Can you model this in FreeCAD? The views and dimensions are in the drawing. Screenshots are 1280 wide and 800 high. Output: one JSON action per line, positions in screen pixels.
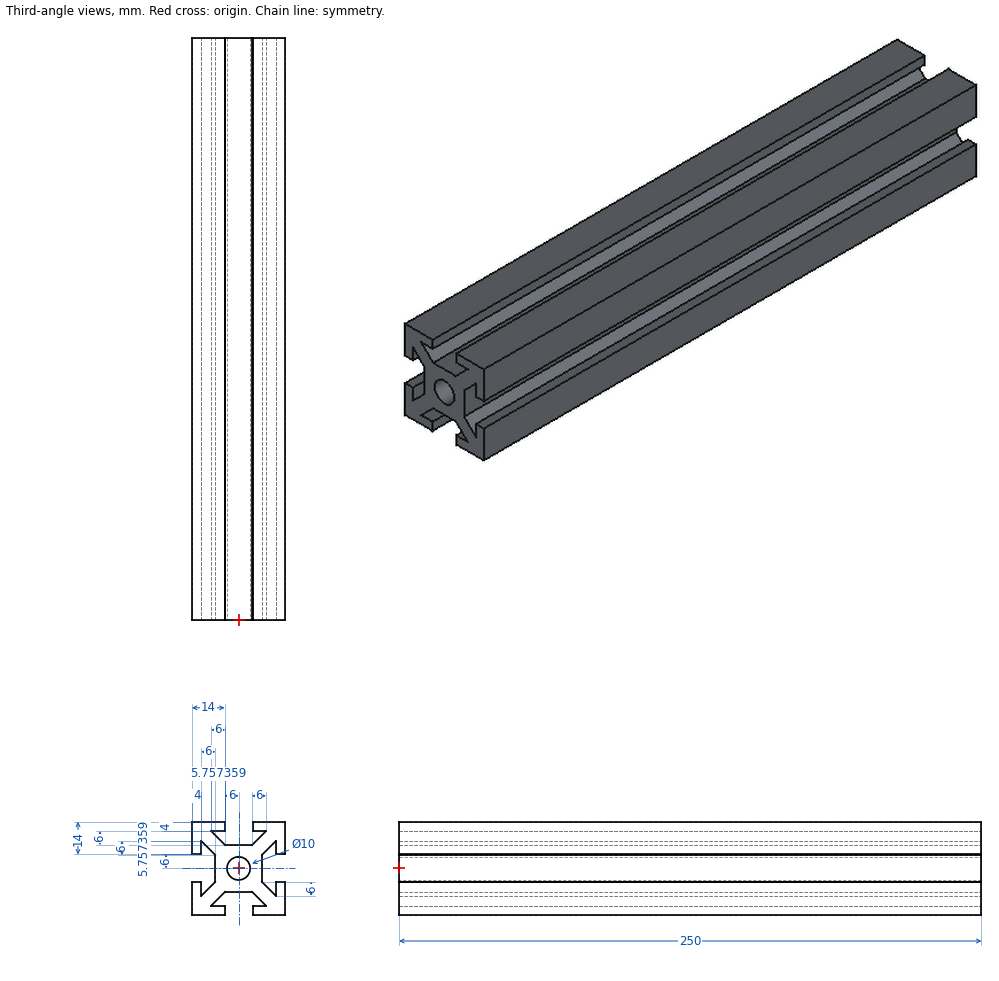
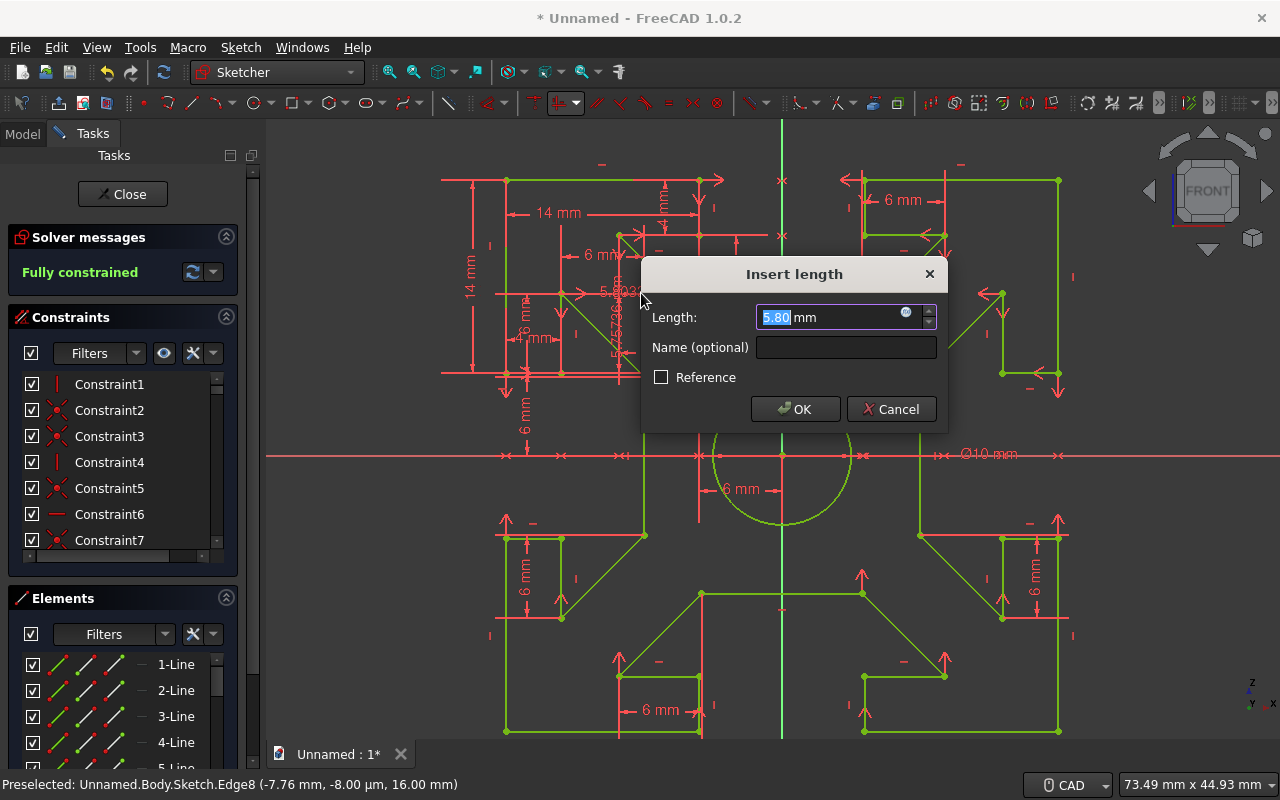
{"action": "type", "text": "5.757359"}
{"action": "key", "text": "Return"}
{"action": "key", "text": "Escape"}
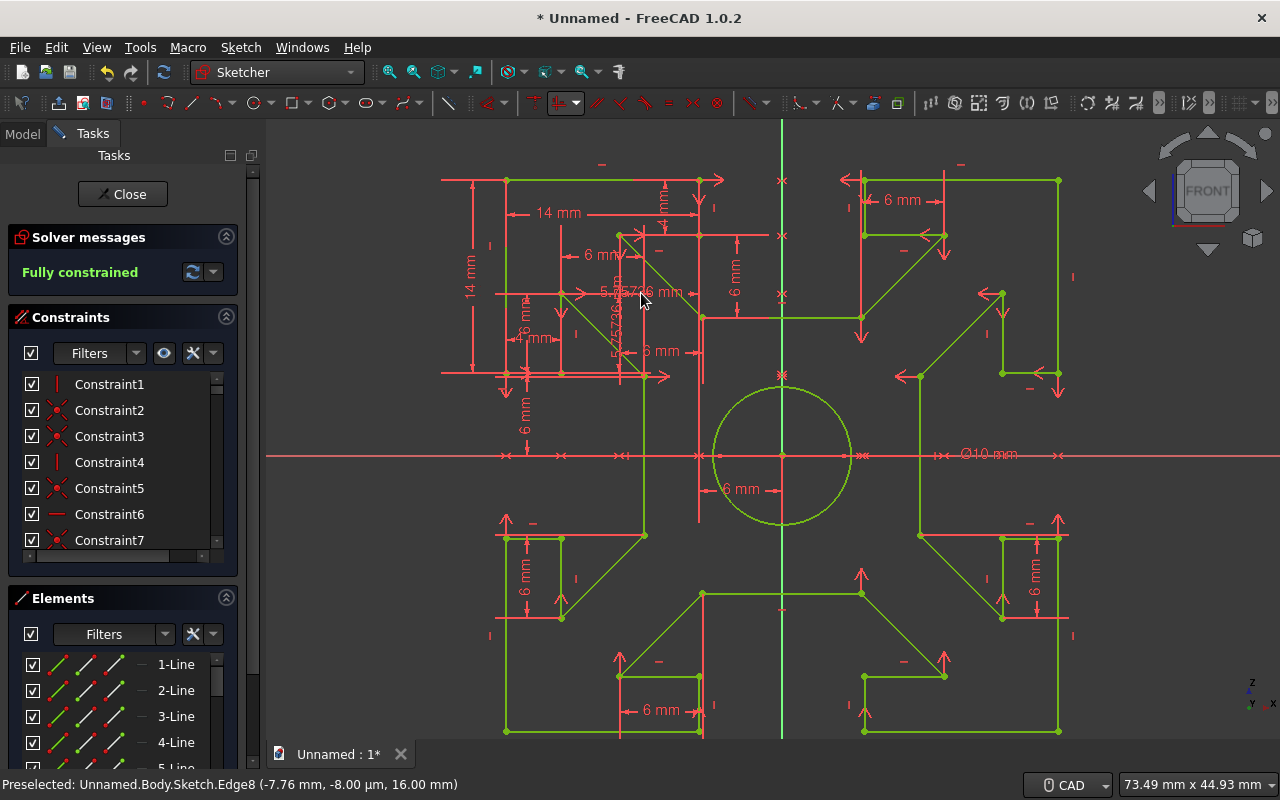
{"action": "left_click", "coordinate": [123, 194]}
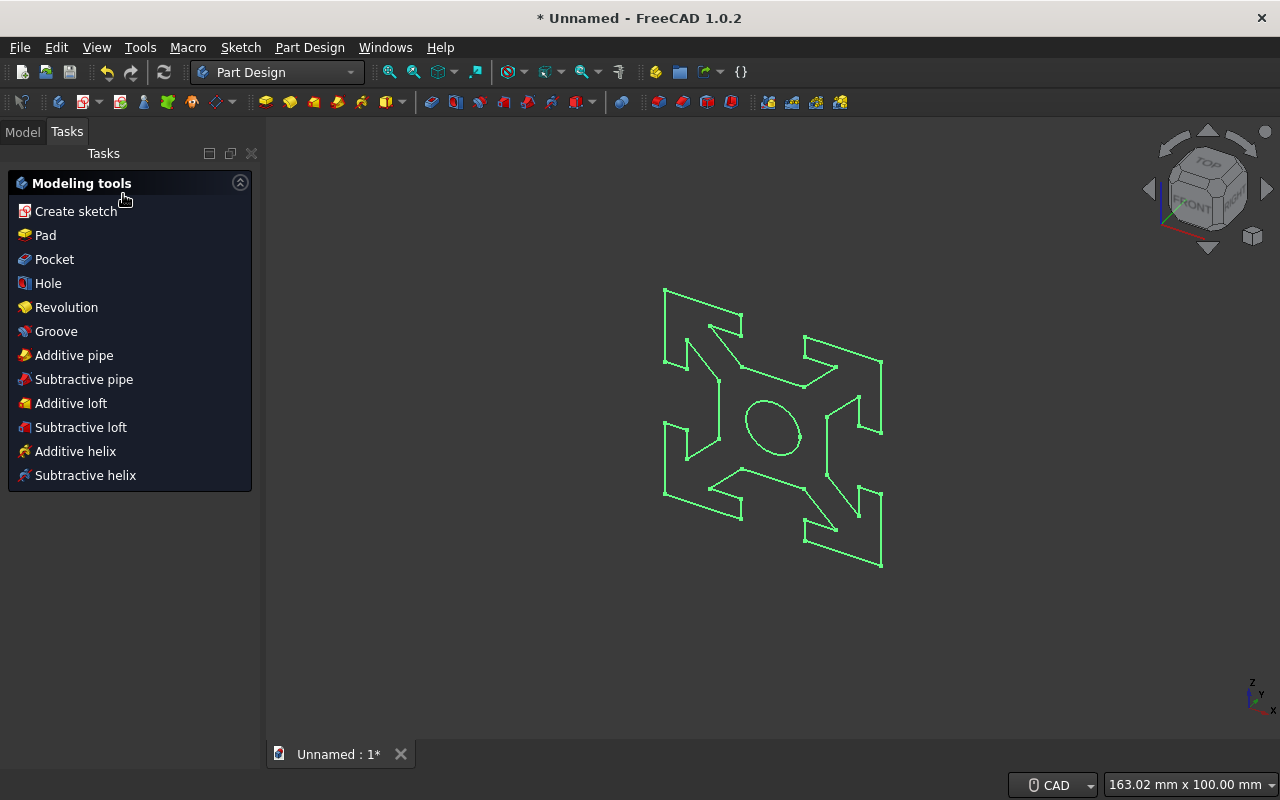
{"action": "left_click", "coordinate": [266, 102]}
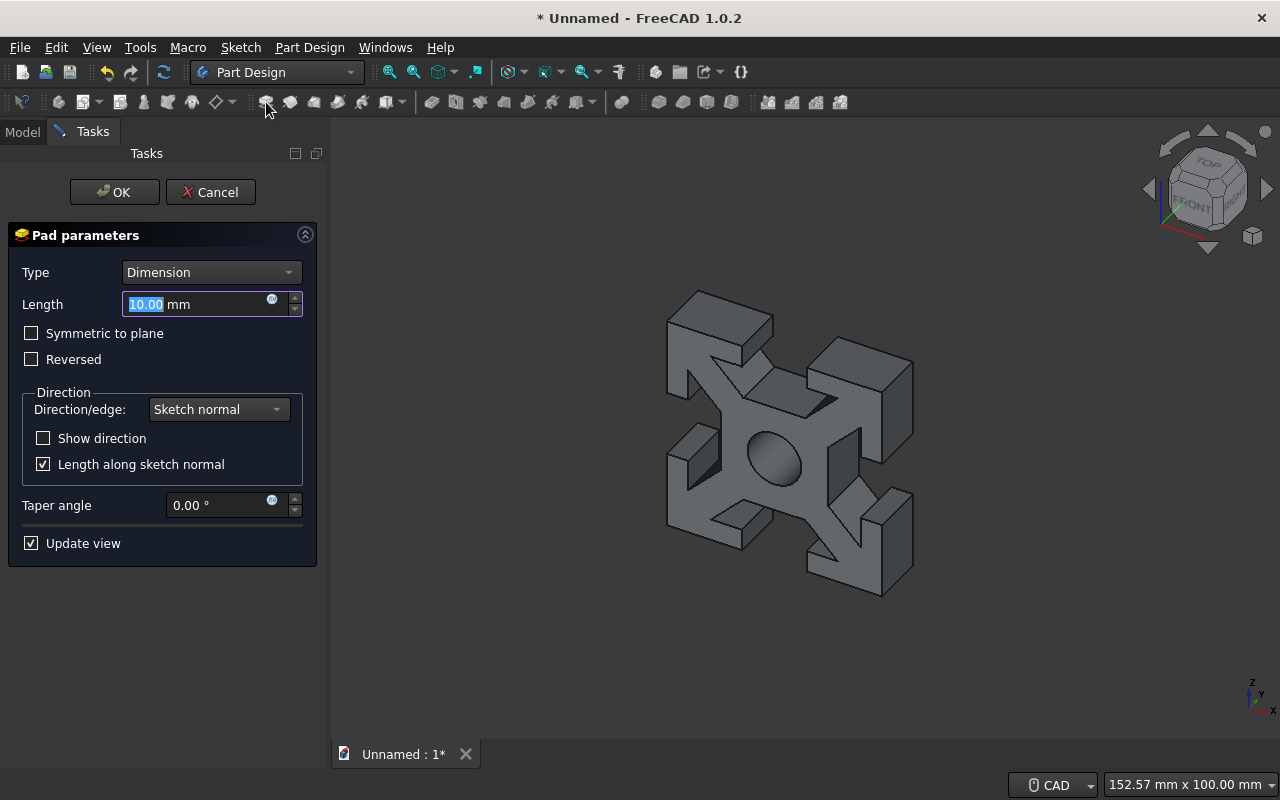
{"action": "type", "text": "250"}
{"action": "key", "text": "Tab"}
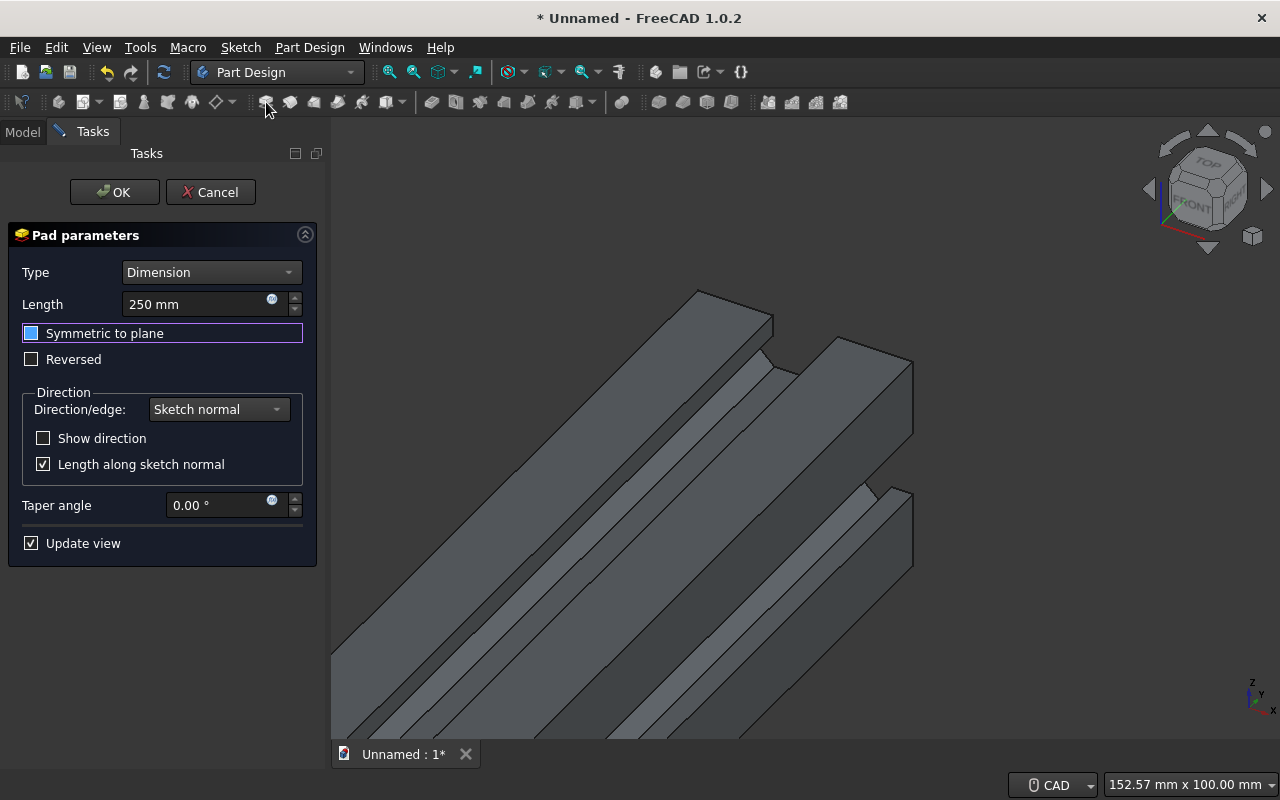
{"action": "left_click", "coordinate": [30, 359]}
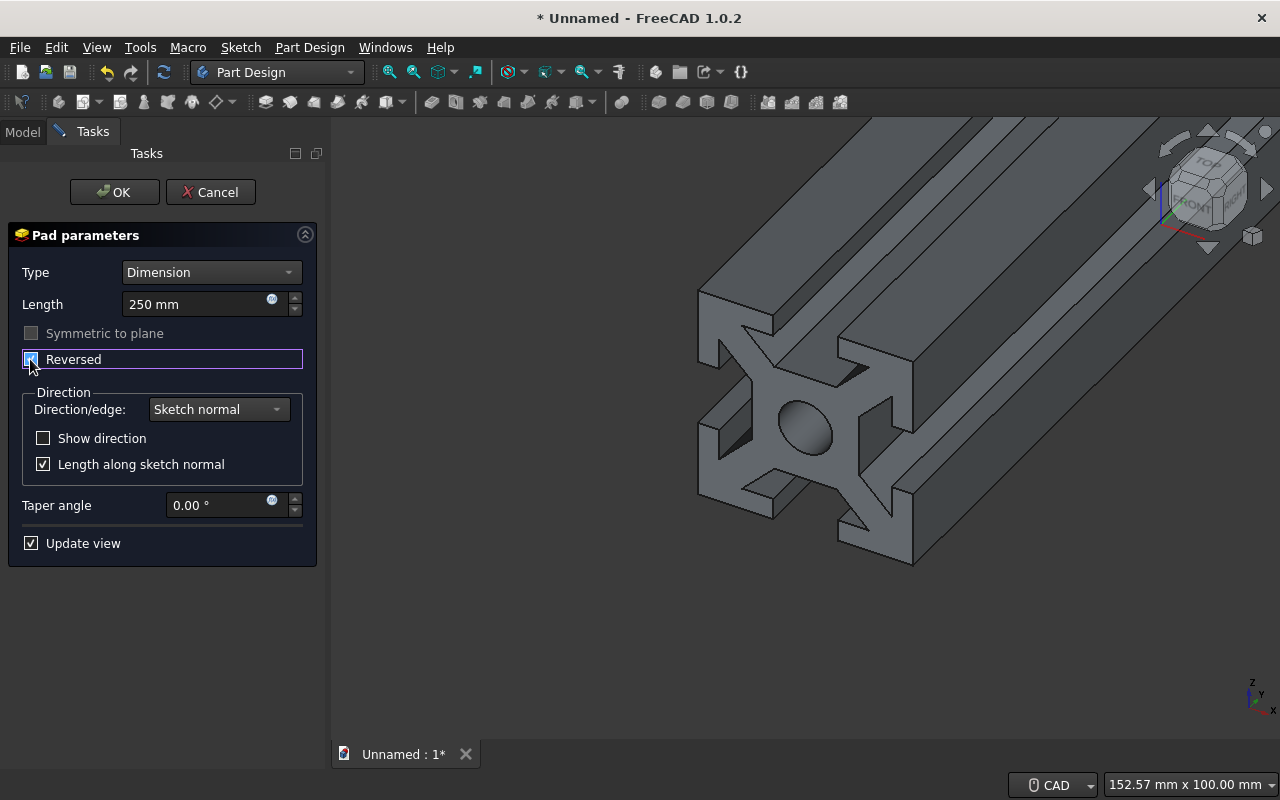
{"action": "left_click", "coordinate": [115, 192]}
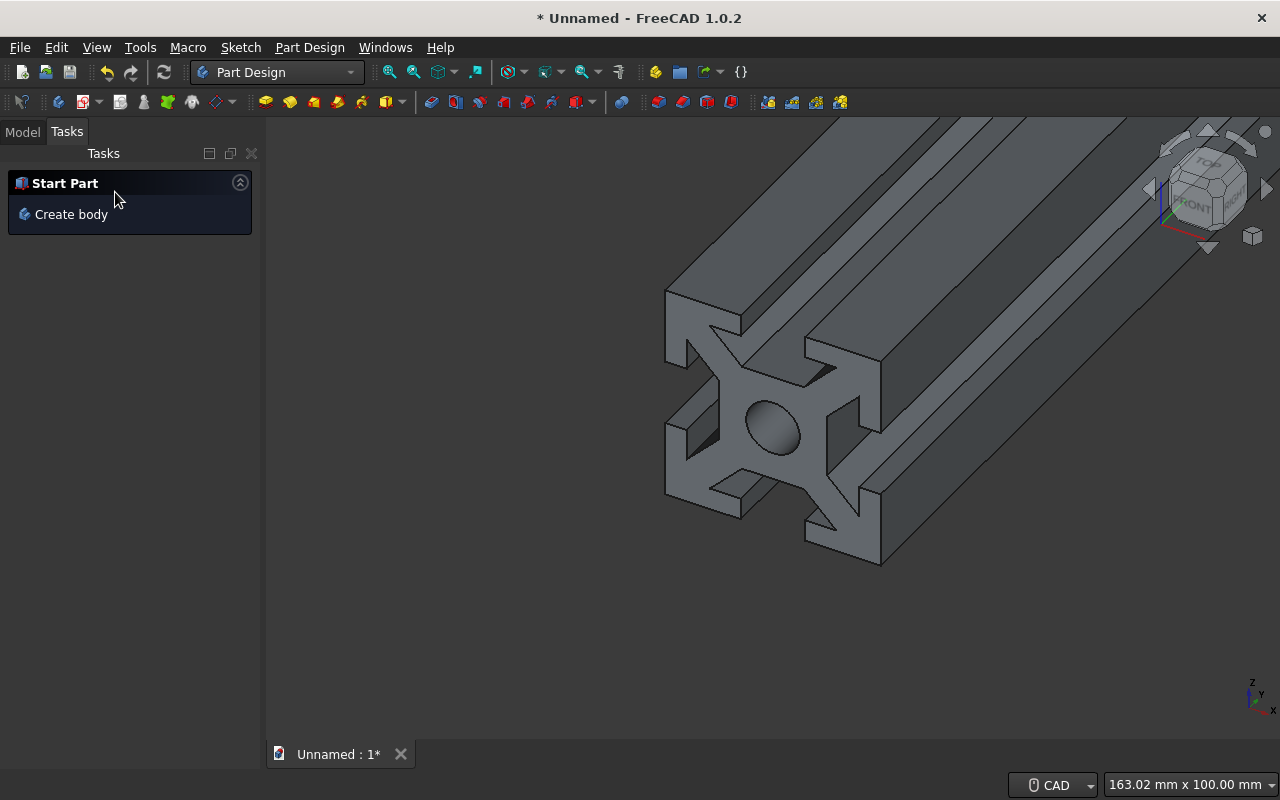
{"action": "key", "text": "0"}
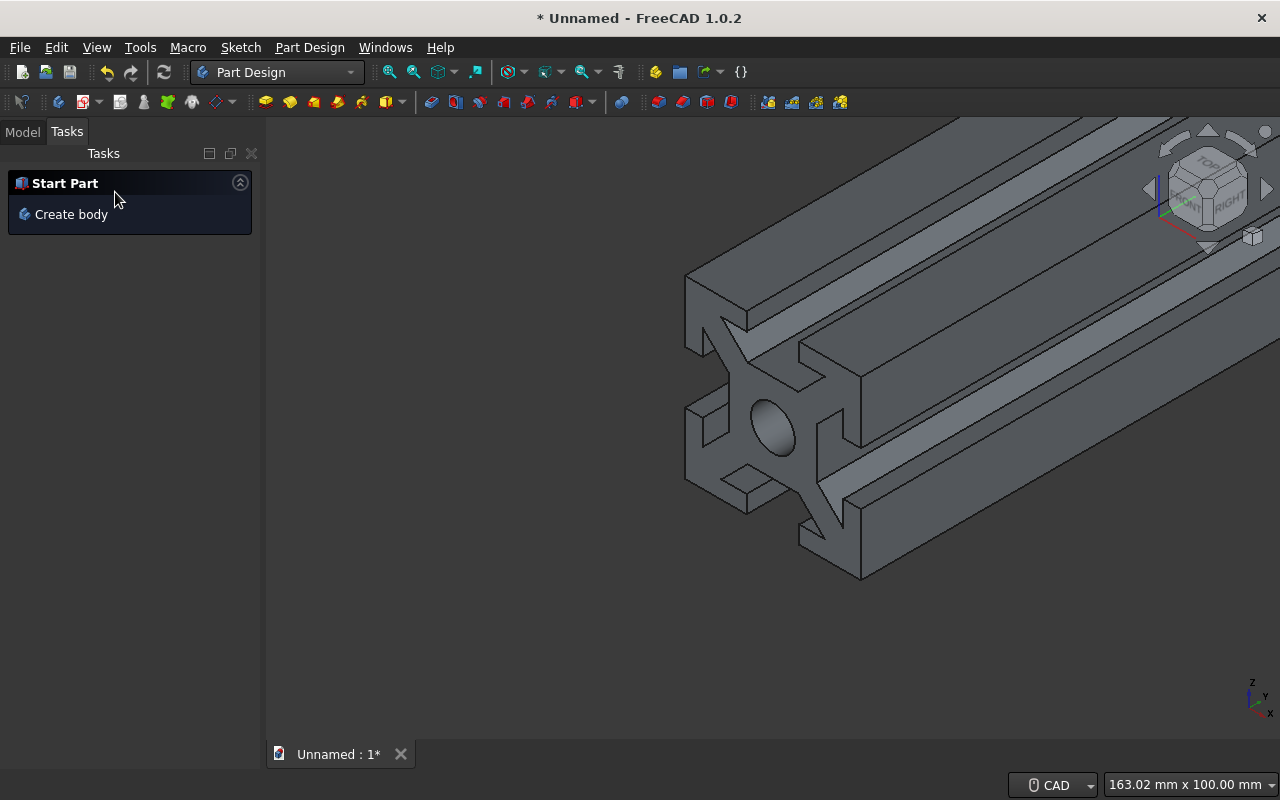
{"action": "left_click", "coordinate": [390, 72]}